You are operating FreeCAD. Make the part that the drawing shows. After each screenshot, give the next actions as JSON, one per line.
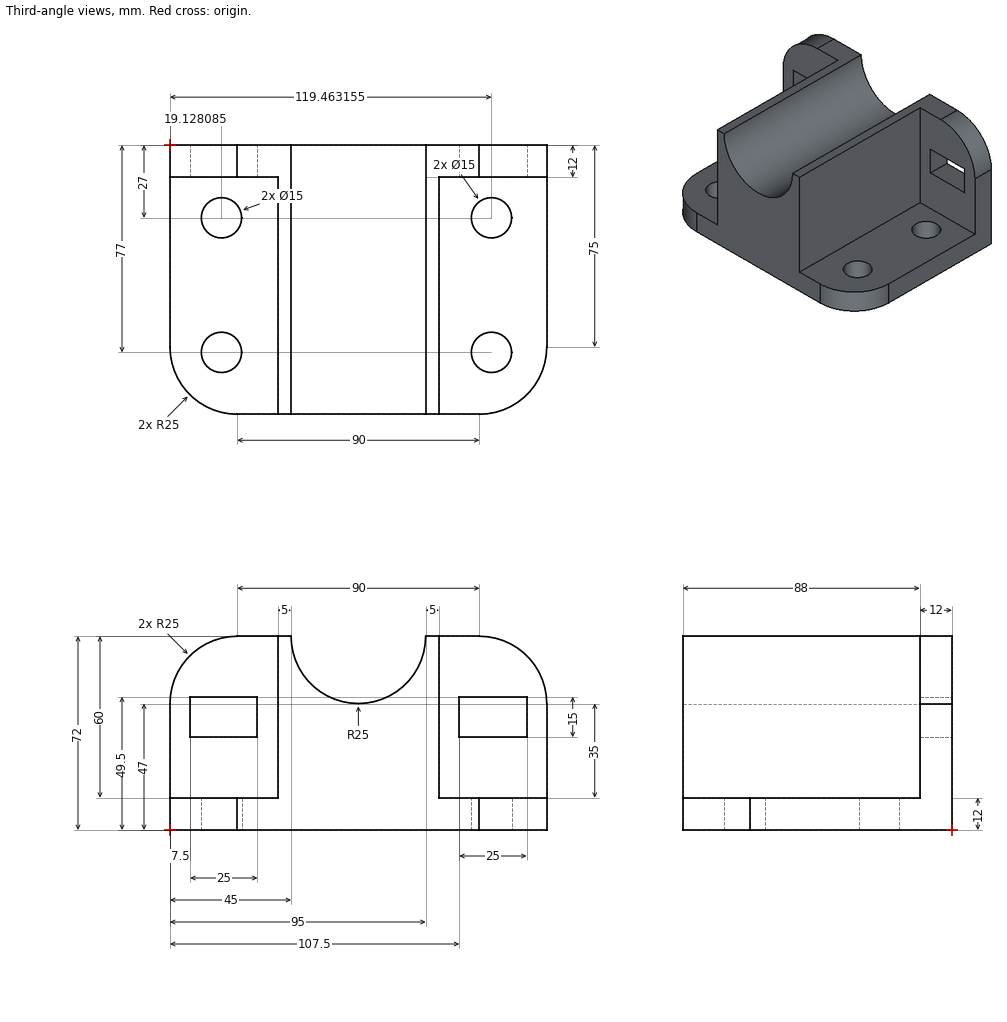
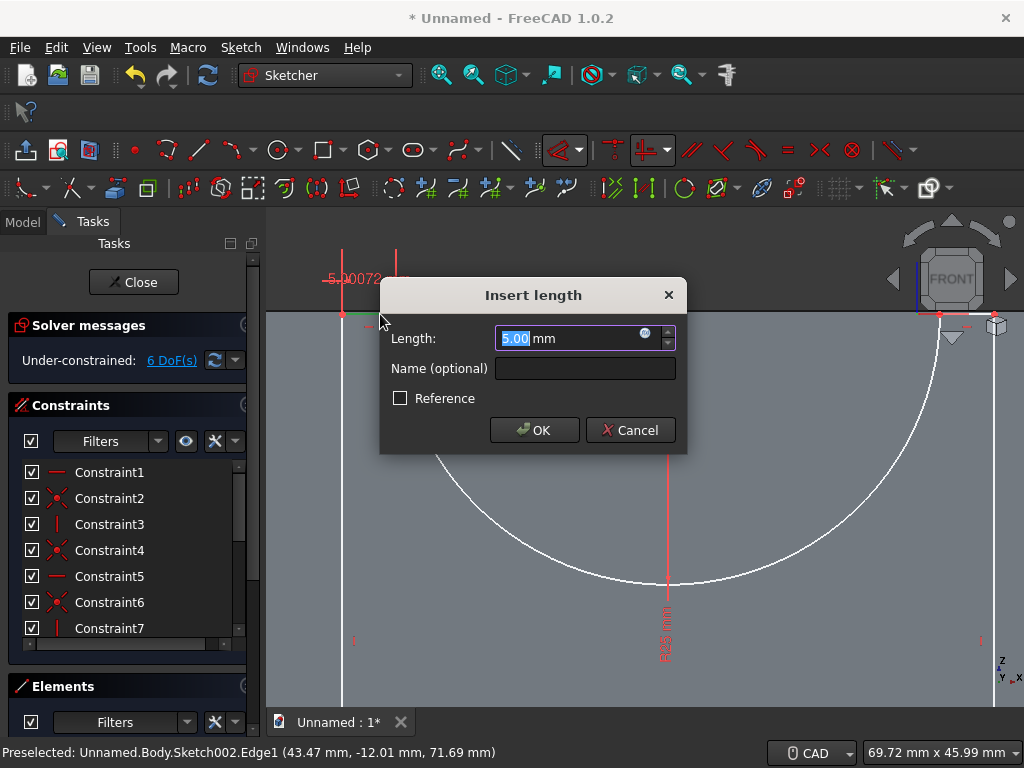
{"action": "type", "text": "5"}
{"action": "key", "text": "Return"}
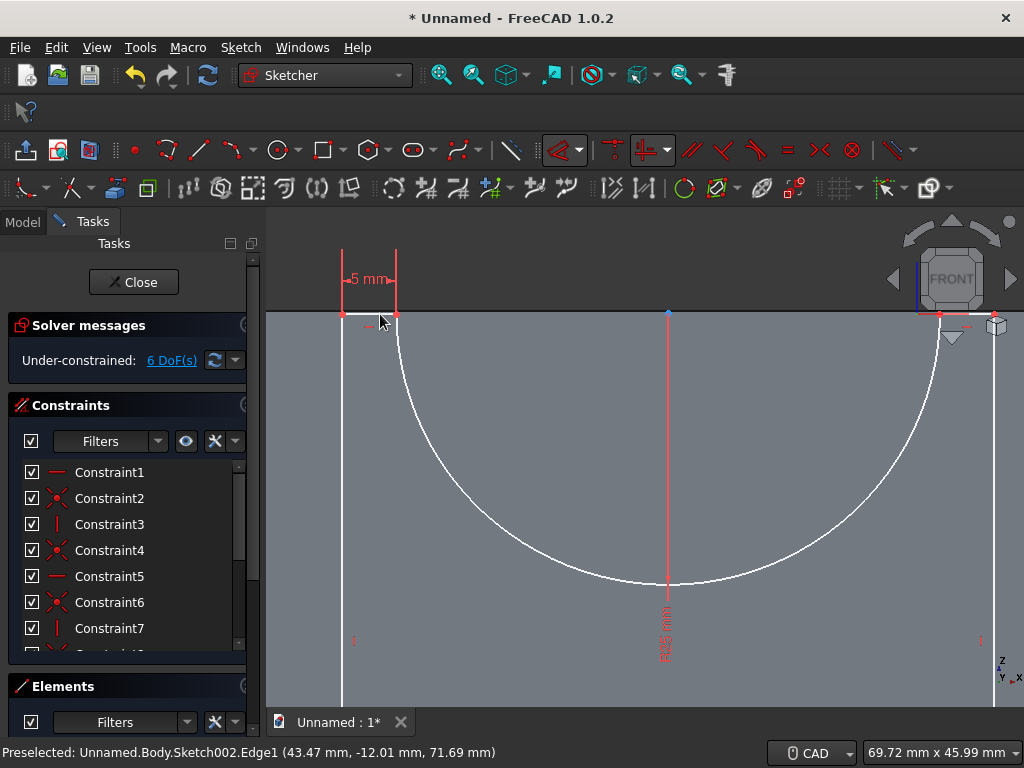
{"action": "scroll", "coordinate": [650, 314], "scroll_direction": "down", "scroll_amount": 5}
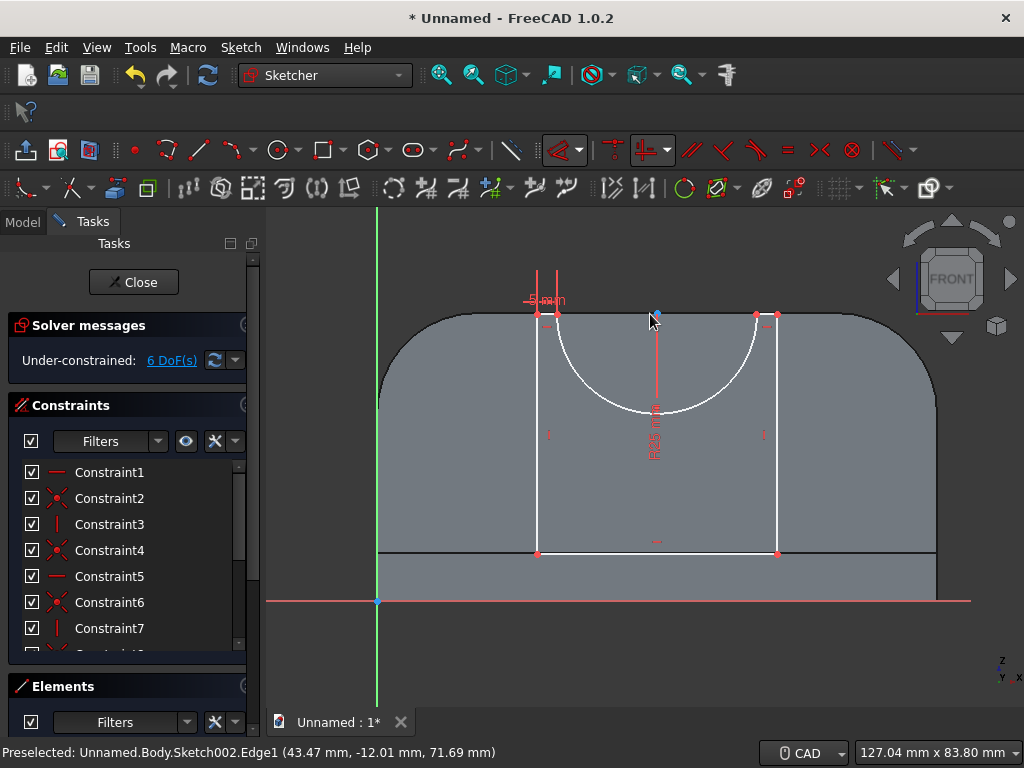
{"action": "scroll", "coordinate": [771, 314], "scroll_direction": "up", "scroll_amount": 5}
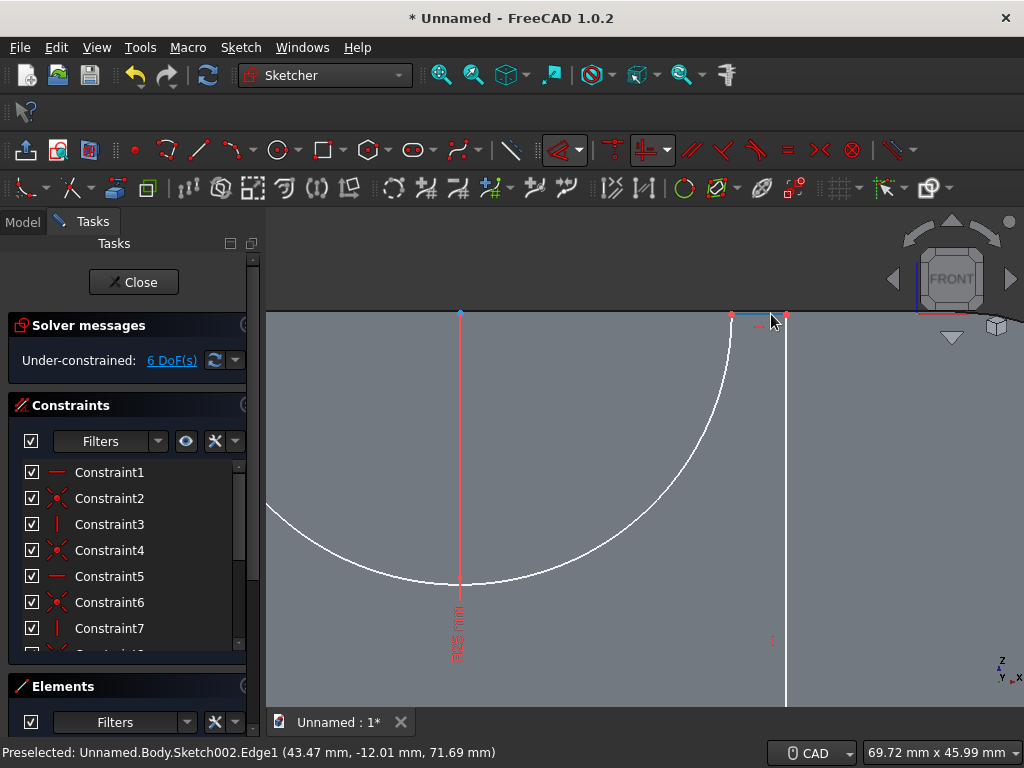
{"action": "left_click", "coordinate": [770, 314]}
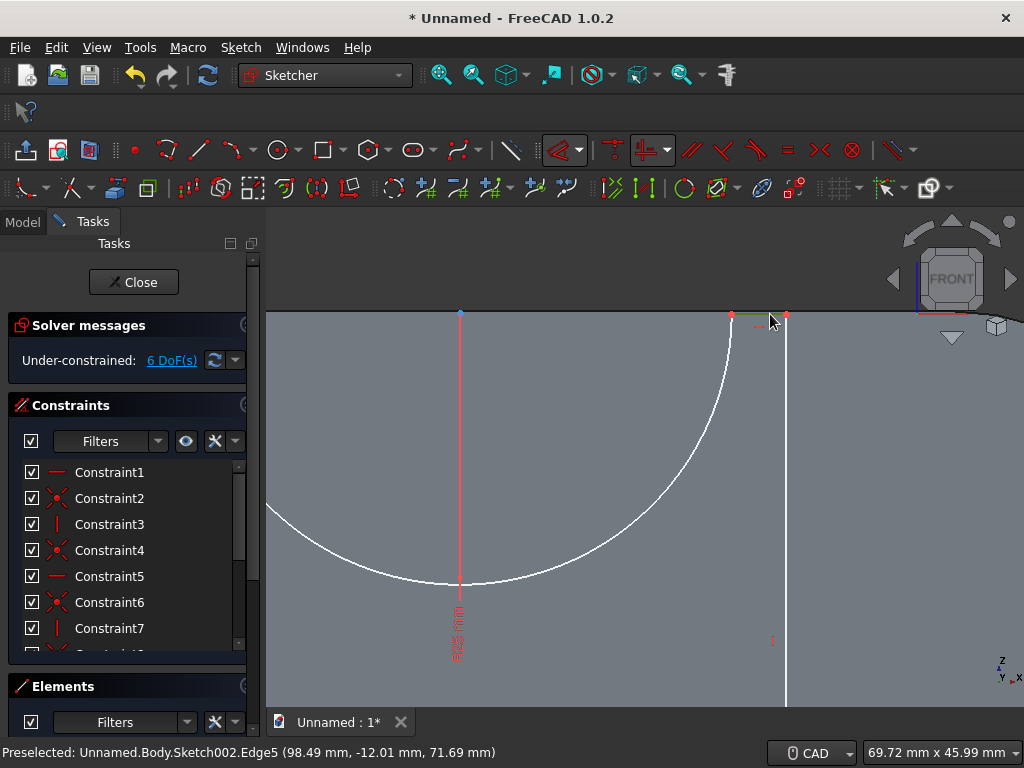
{"action": "left_click", "coordinate": [582, 150]}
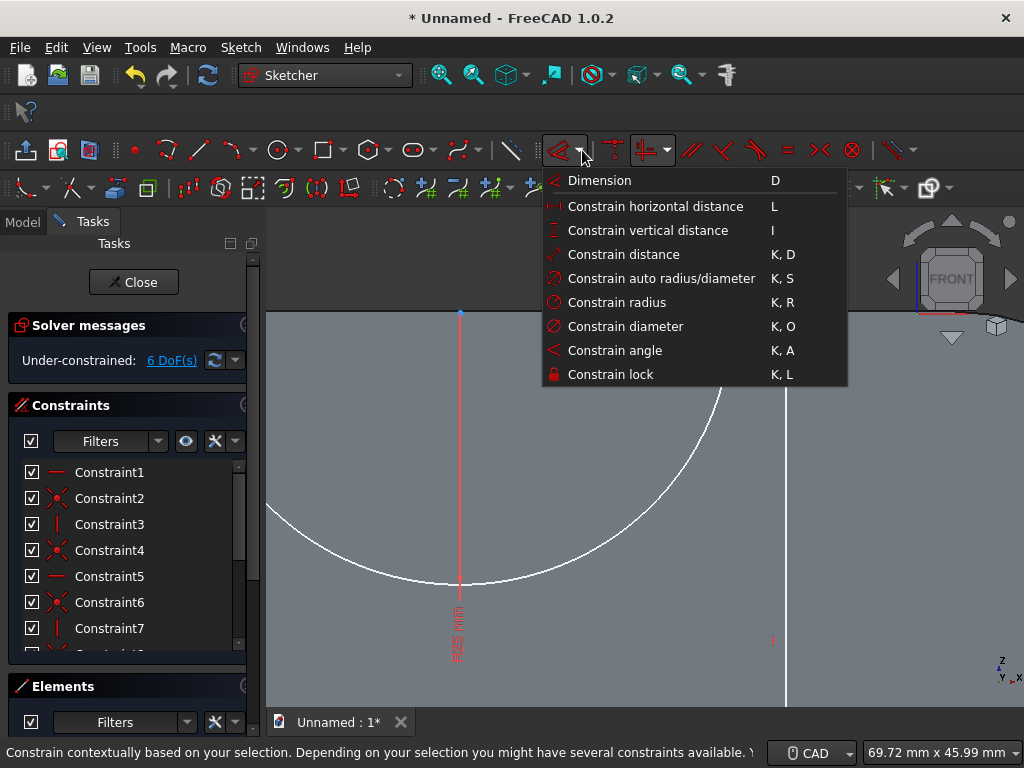
{"action": "left_click", "coordinate": [695, 206]}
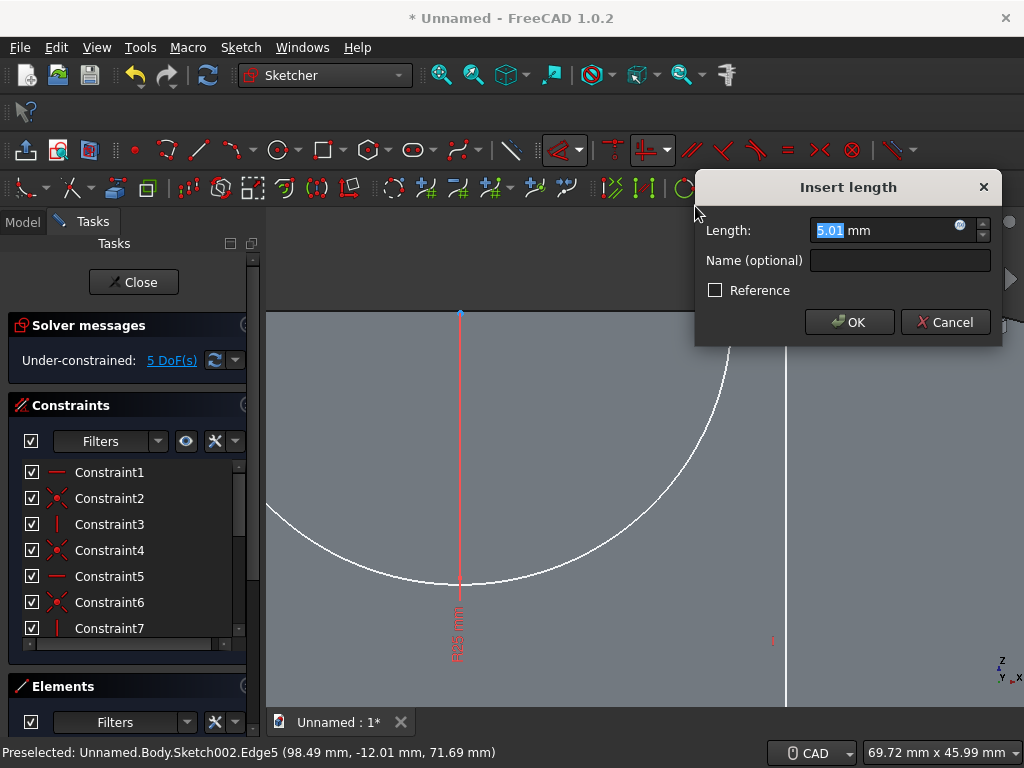
{"action": "type", "text": "5"}
{"action": "key", "text": "Return"}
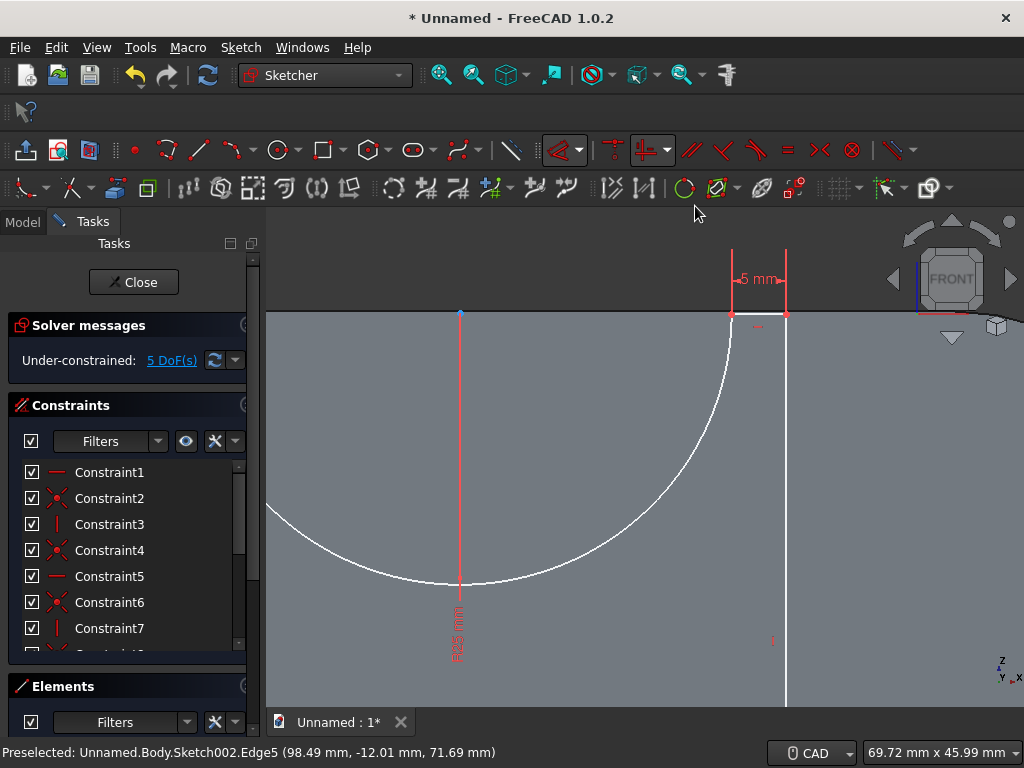
{"action": "scroll", "coordinate": [771, 314], "scroll_direction": "down", "scroll_amount": 5}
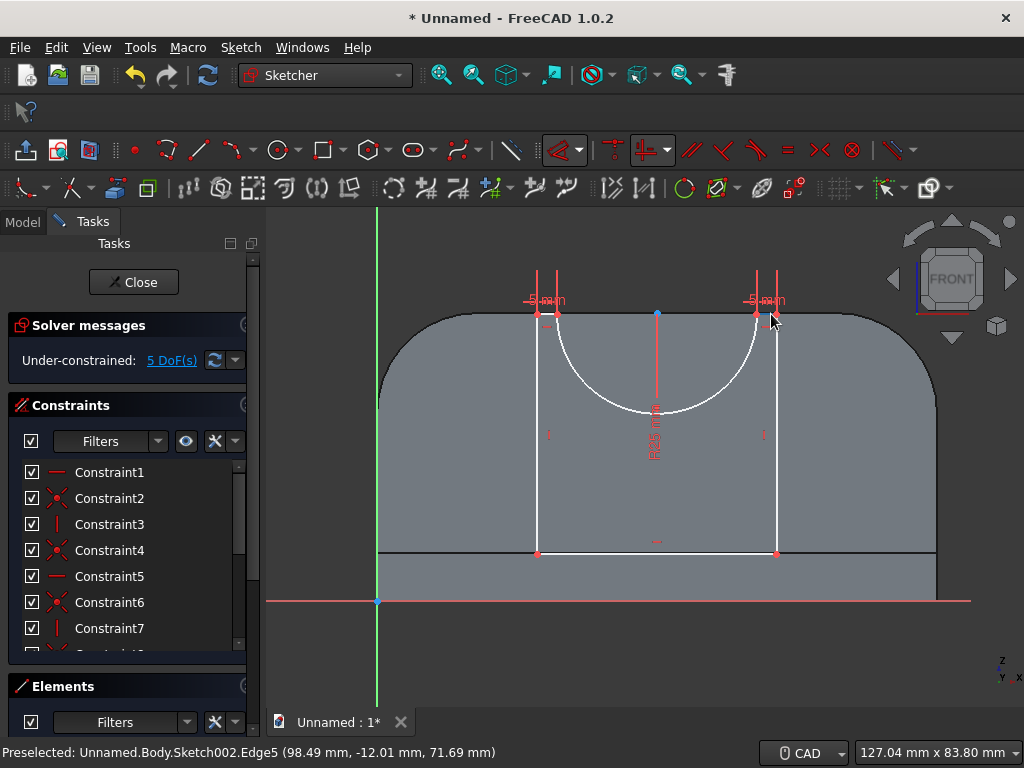
{"action": "left_click", "coordinate": [537, 386]}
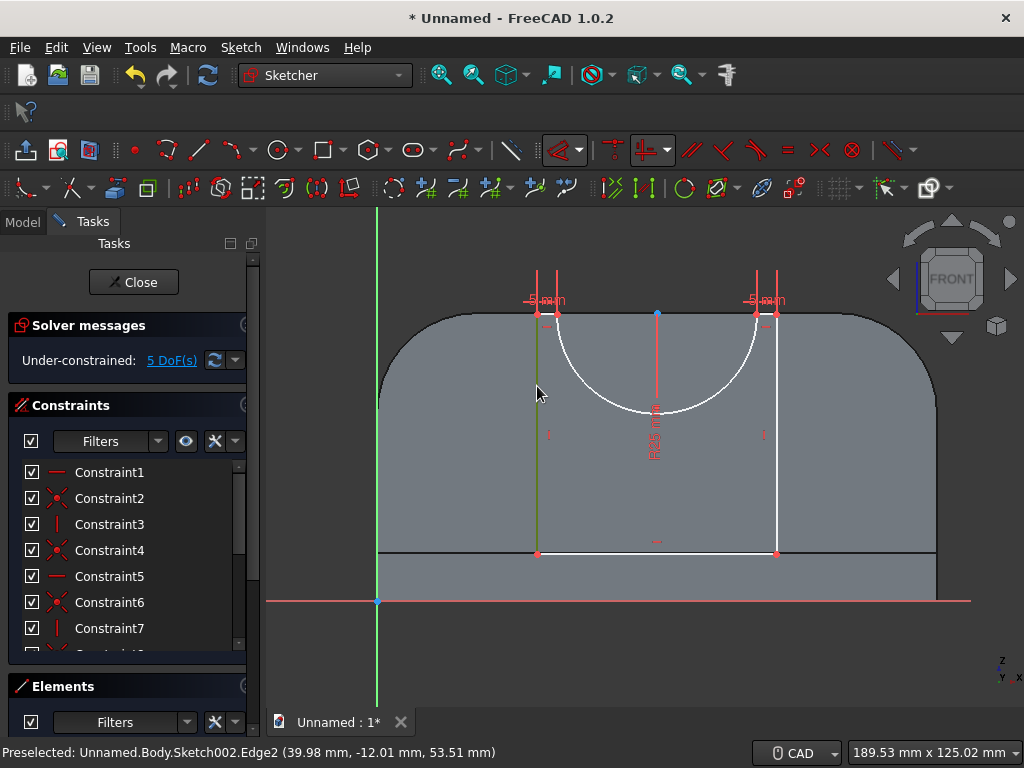
{"action": "left_click", "coordinate": [582, 150]}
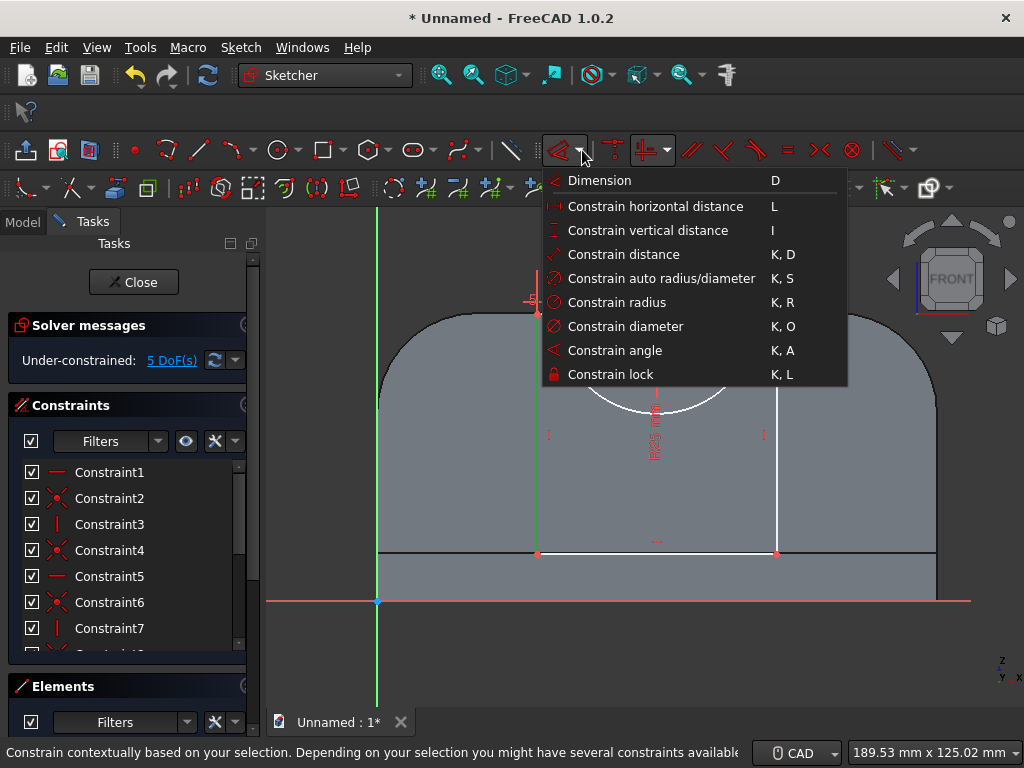
{"action": "left_click", "coordinate": [695, 230]}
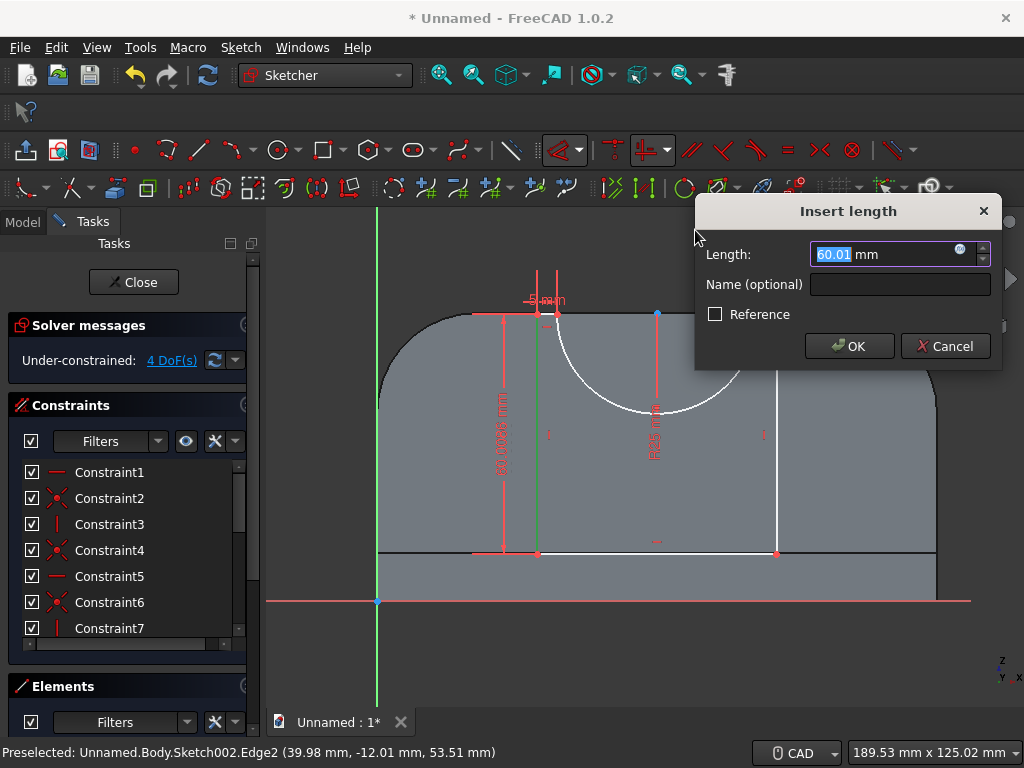
{"action": "type", "text": "60"}
{"action": "key", "text": "Return"}